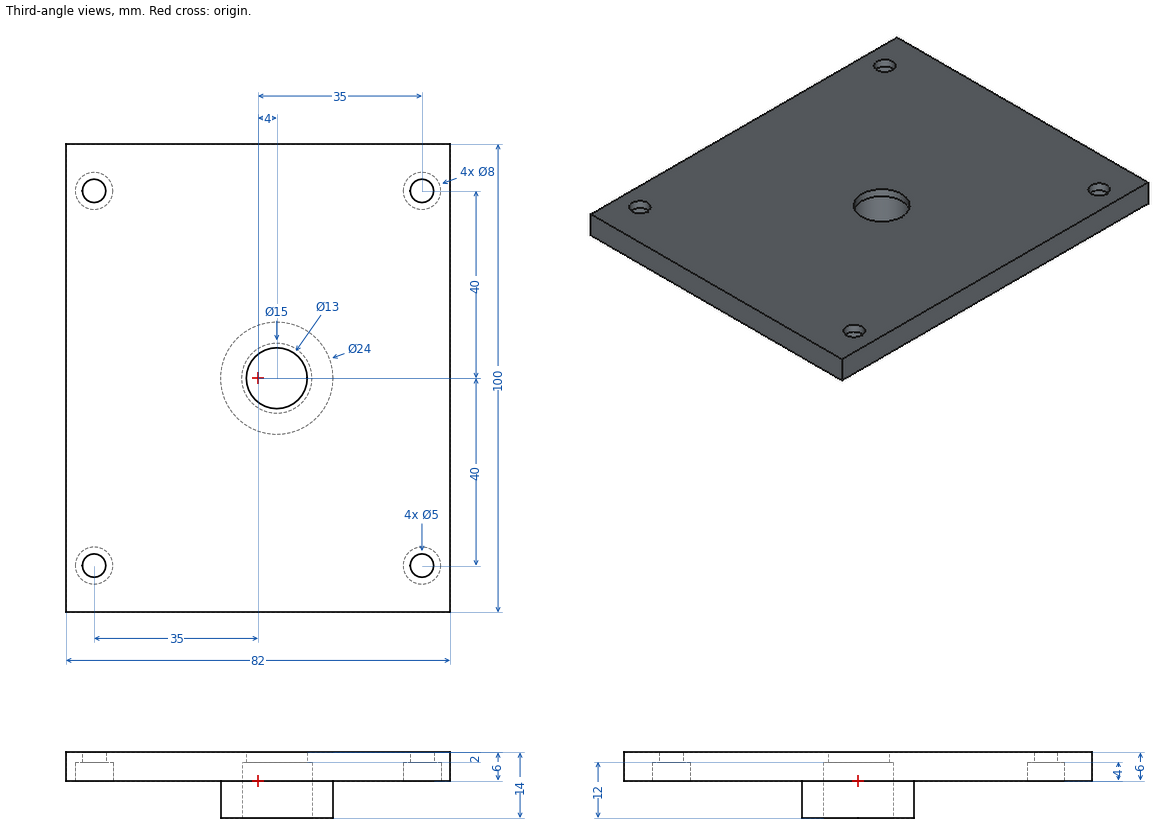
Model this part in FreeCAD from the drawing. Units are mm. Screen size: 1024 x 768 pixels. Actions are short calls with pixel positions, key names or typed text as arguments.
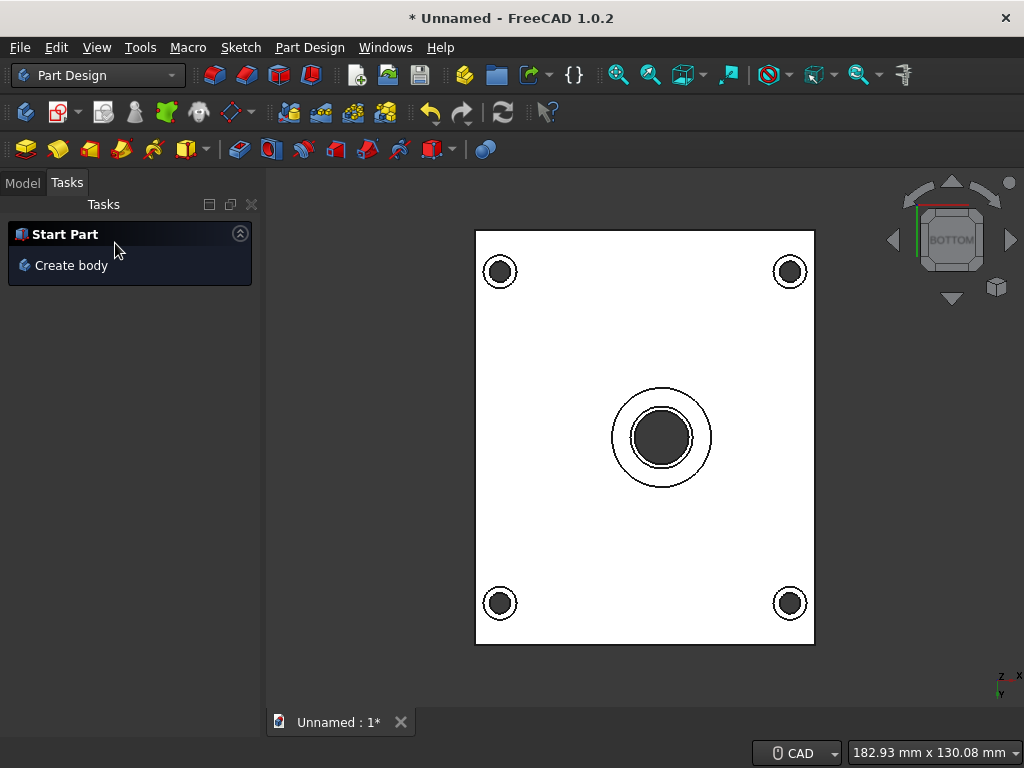
key(0)